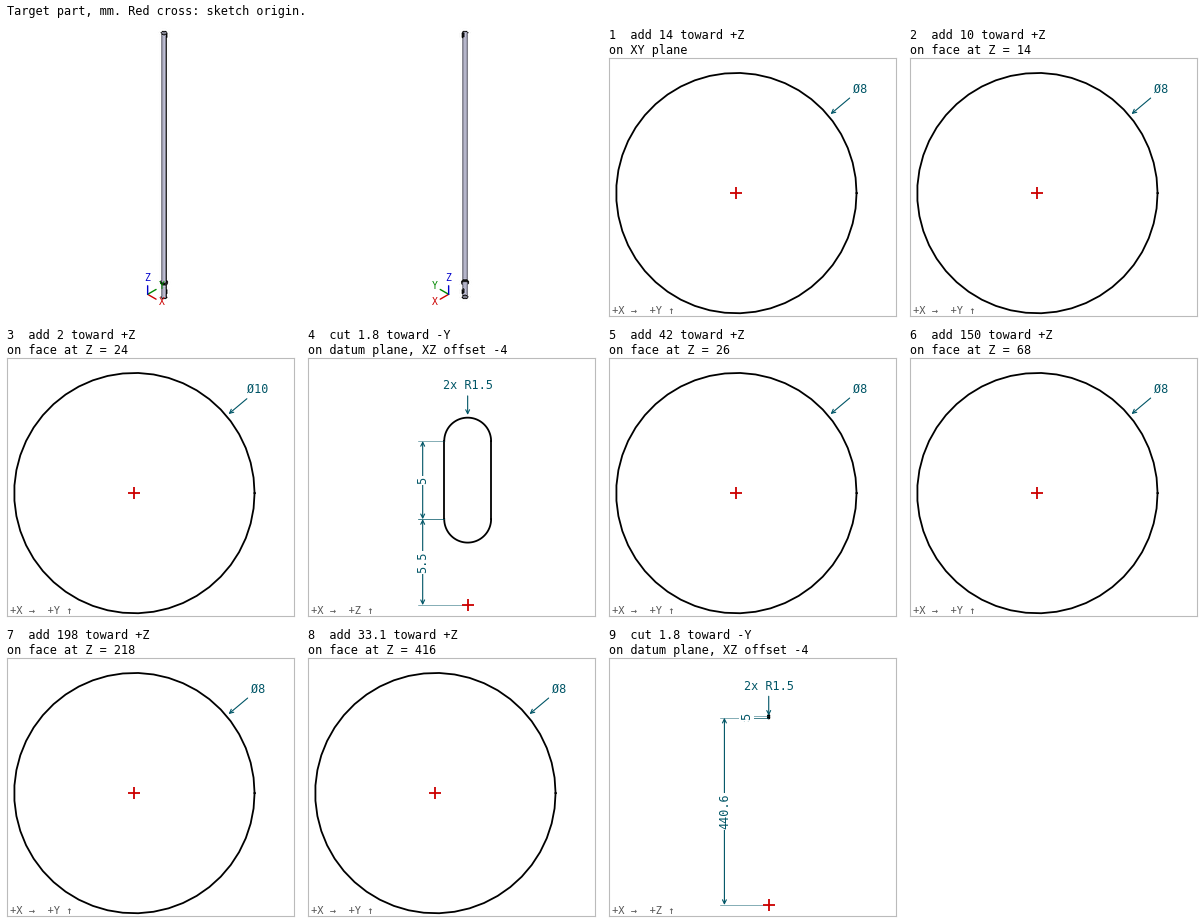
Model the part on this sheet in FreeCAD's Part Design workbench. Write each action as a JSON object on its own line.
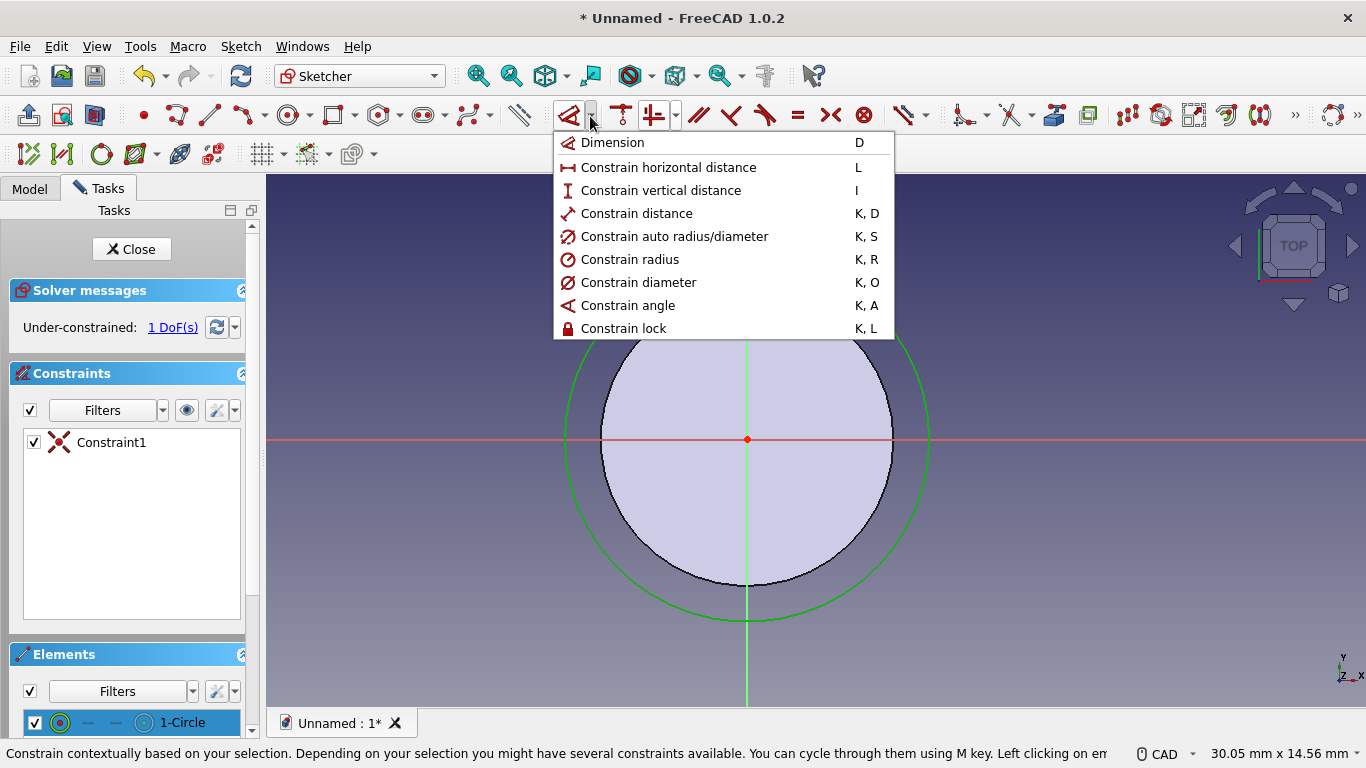
{"action": "left_click", "coordinate": [724, 282]}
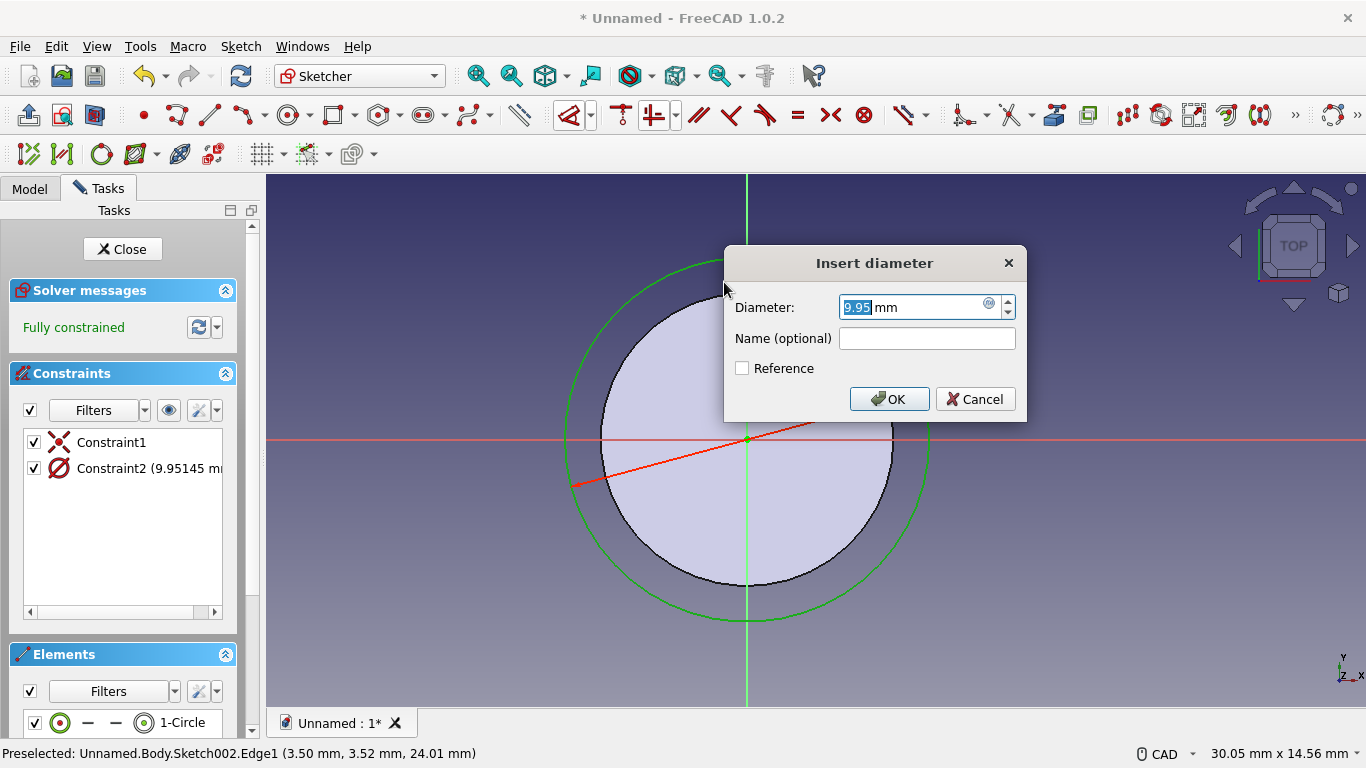
{"action": "type", "text": "10"}
{"action": "key", "text": "Return"}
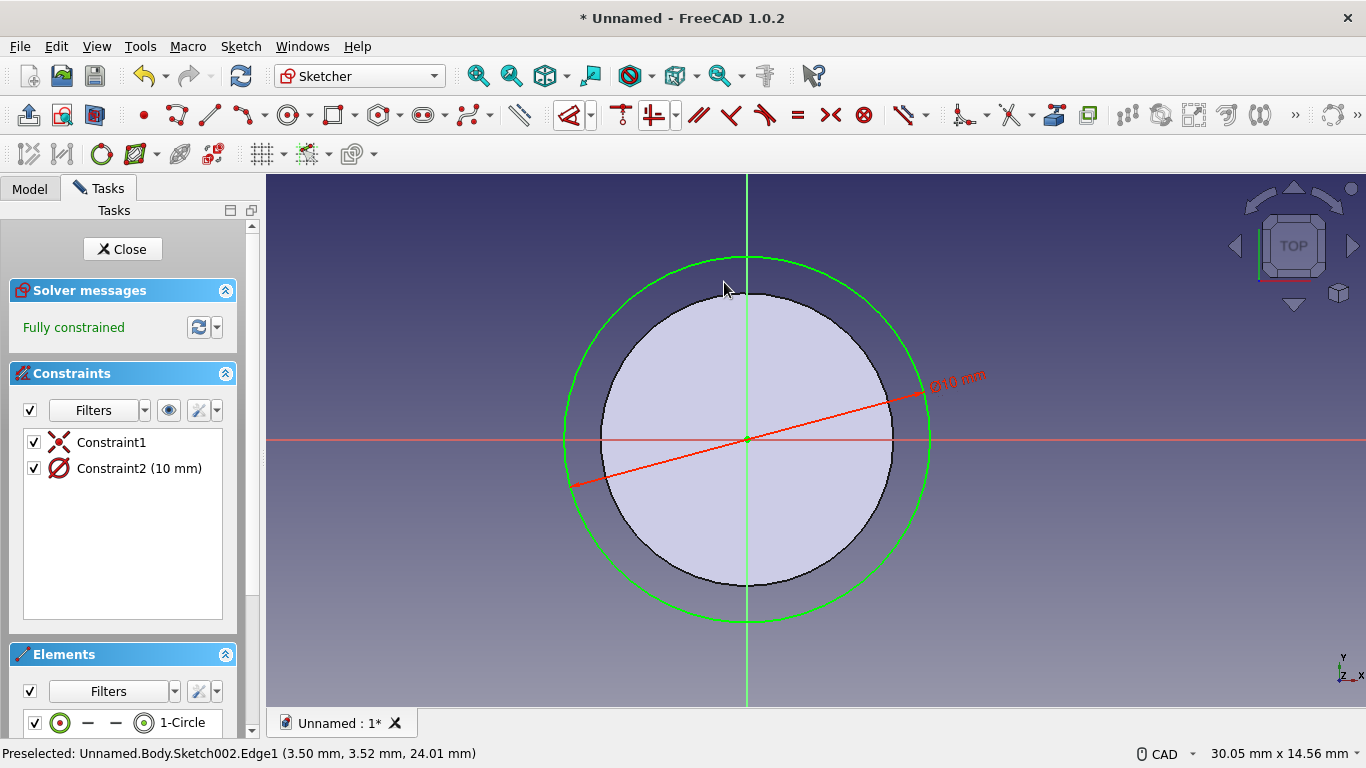
{"action": "left_click", "coordinate": [123, 249]}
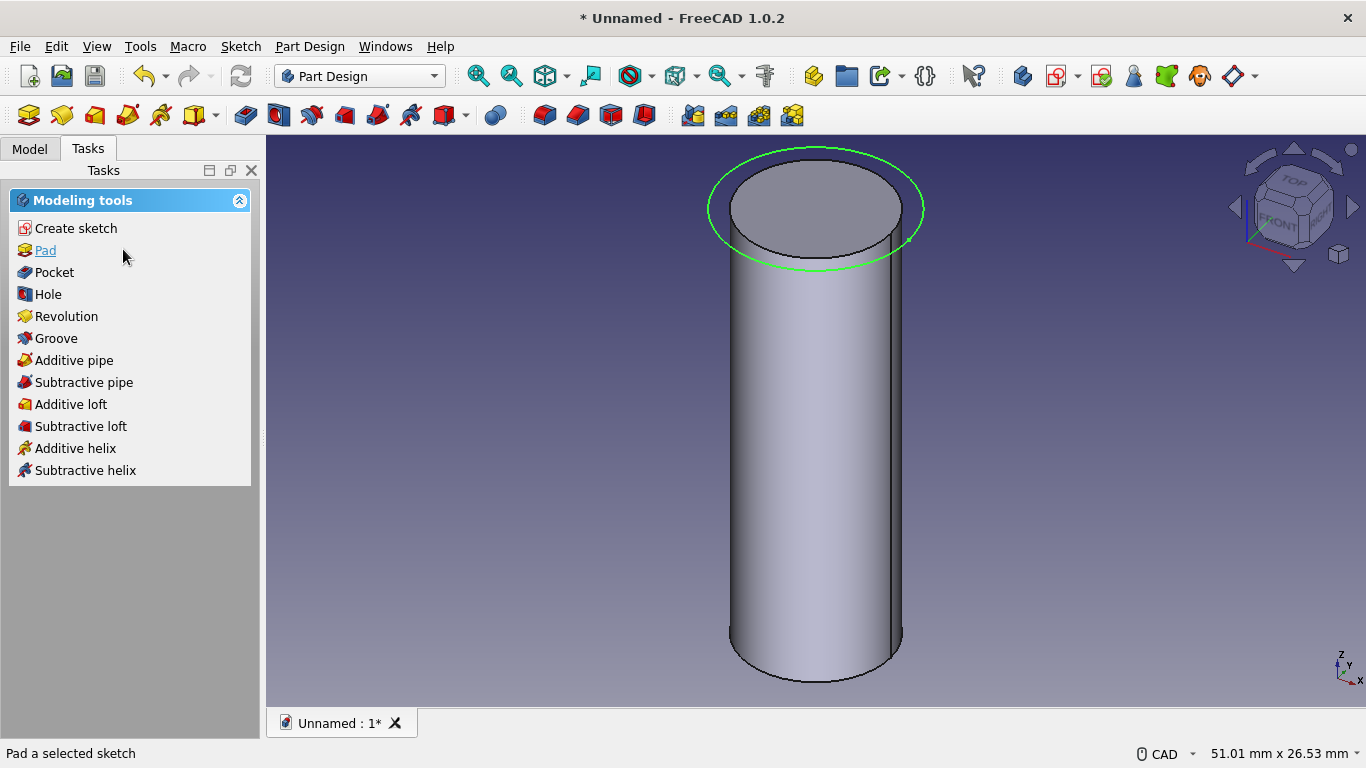
{"action": "left_click", "coordinate": [29, 116]}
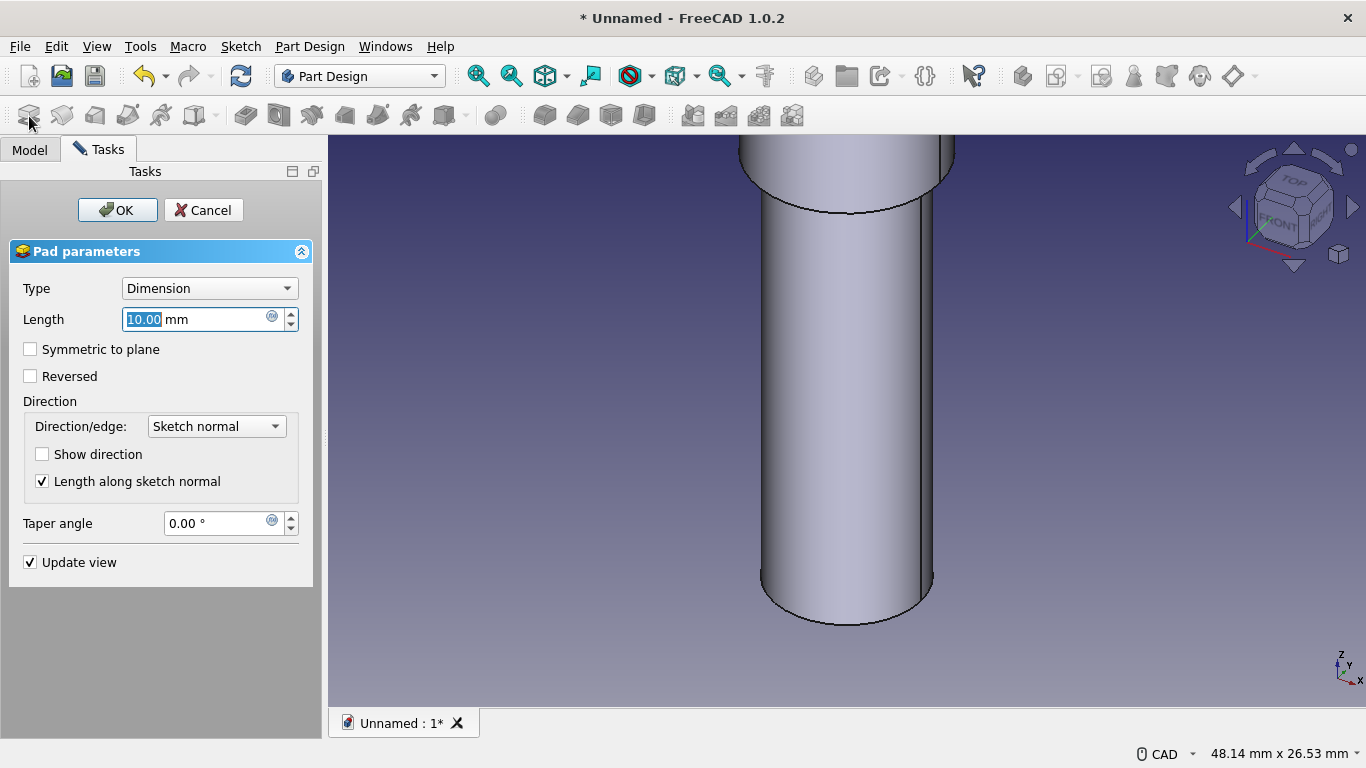
{"action": "type", "text": "2"}
{"action": "key", "text": "Tab"}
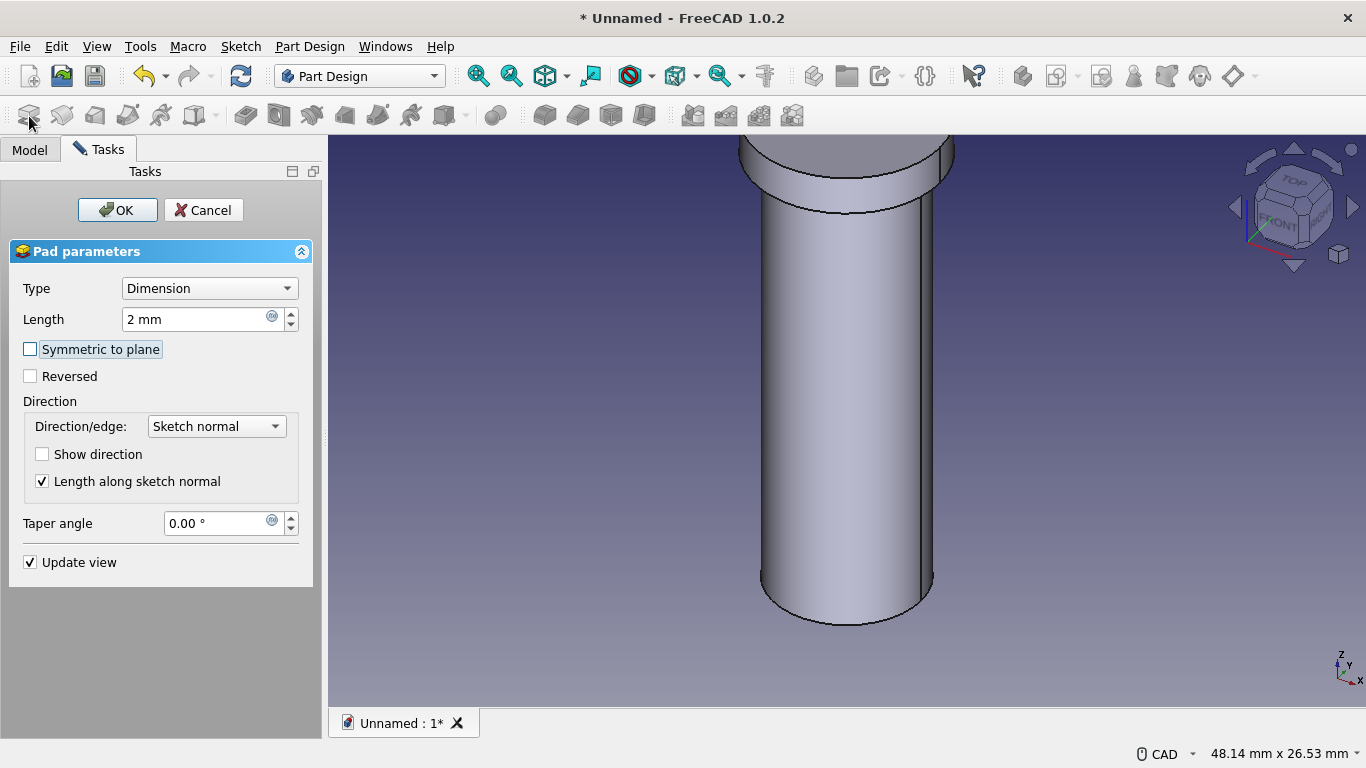
{"action": "left_click", "coordinate": [118, 210]}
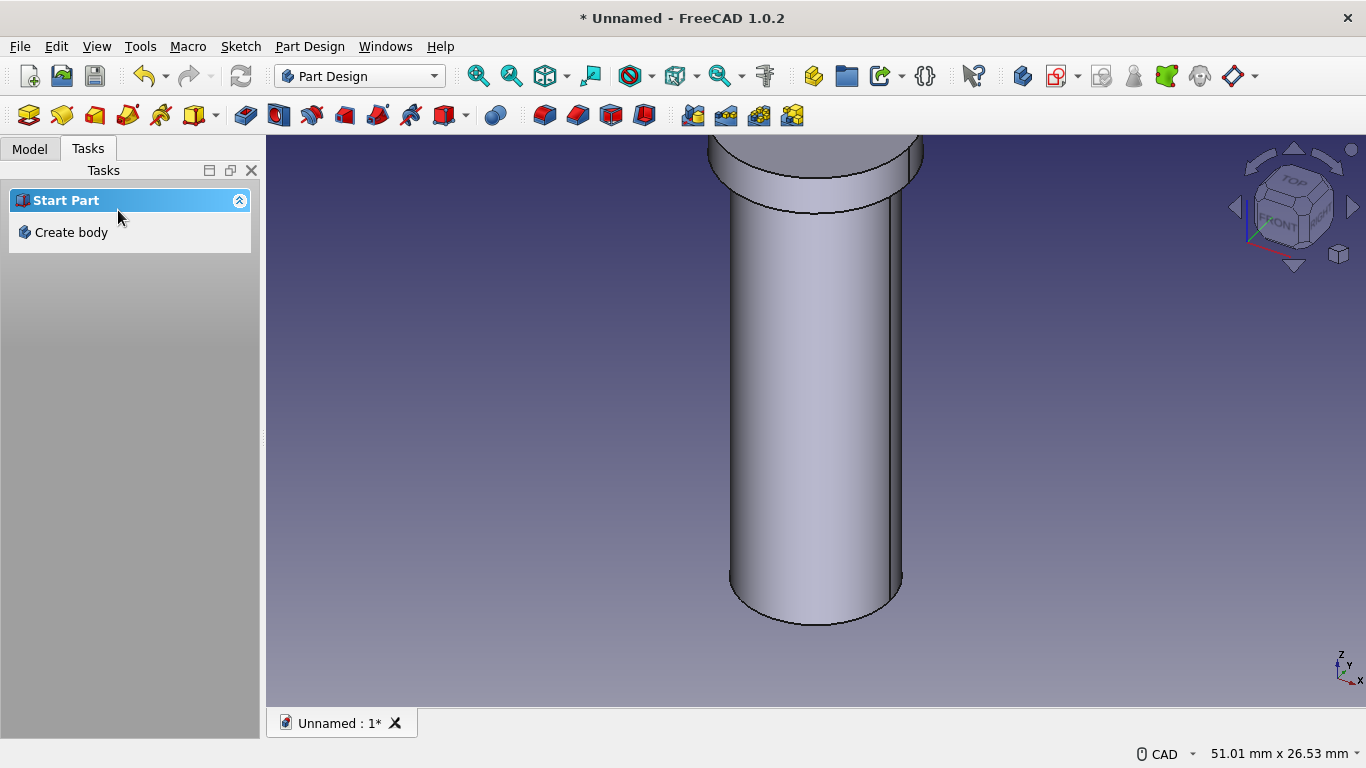
{"action": "left_click", "coordinate": [479, 76]}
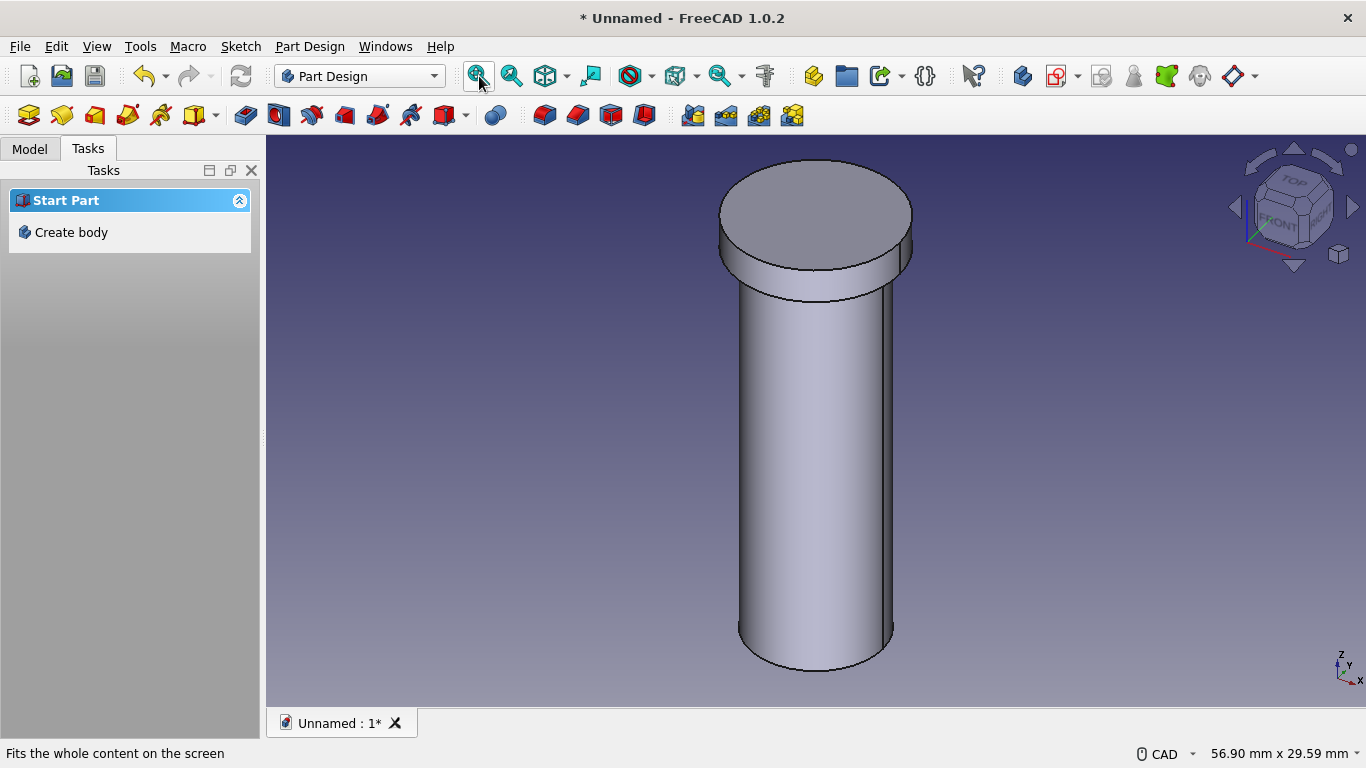
{"action": "left_click", "coordinate": [30, 148]}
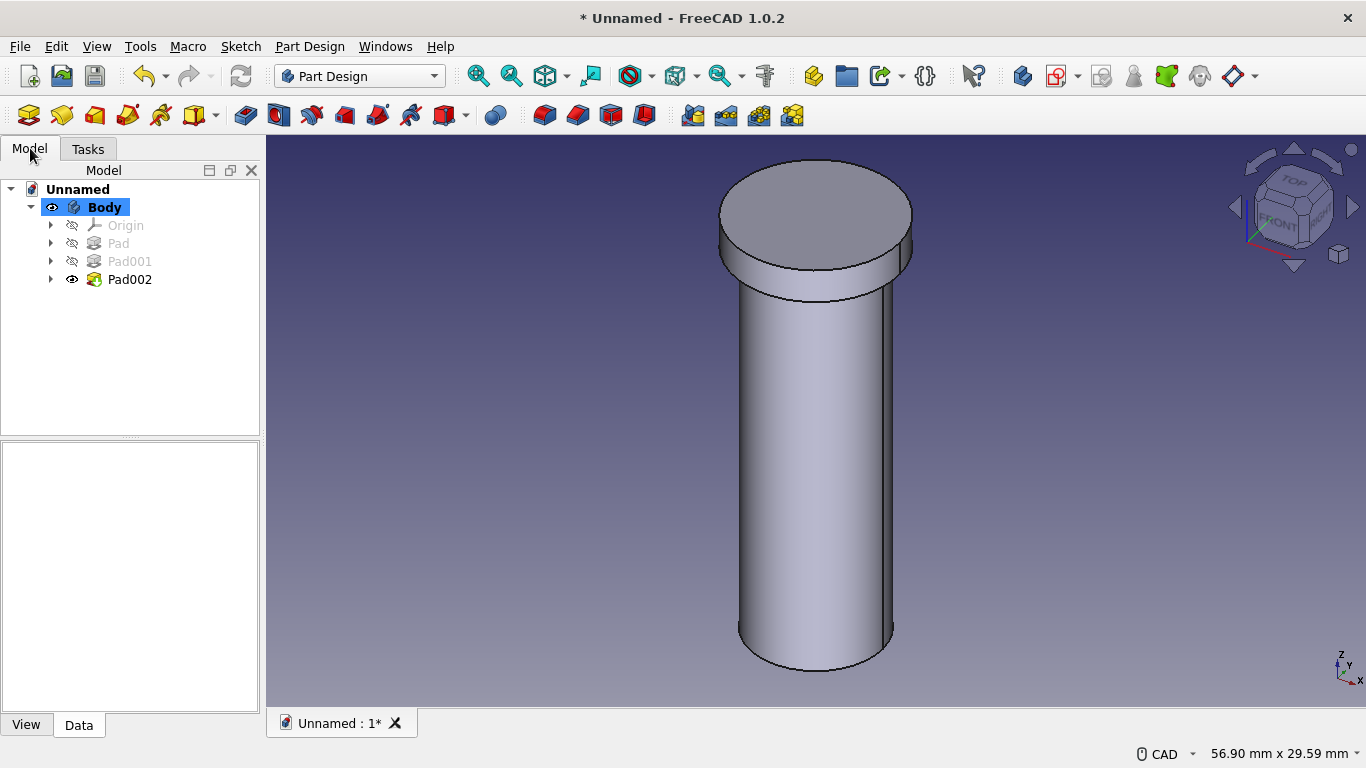
{"action": "left_click", "coordinate": [51, 225]}